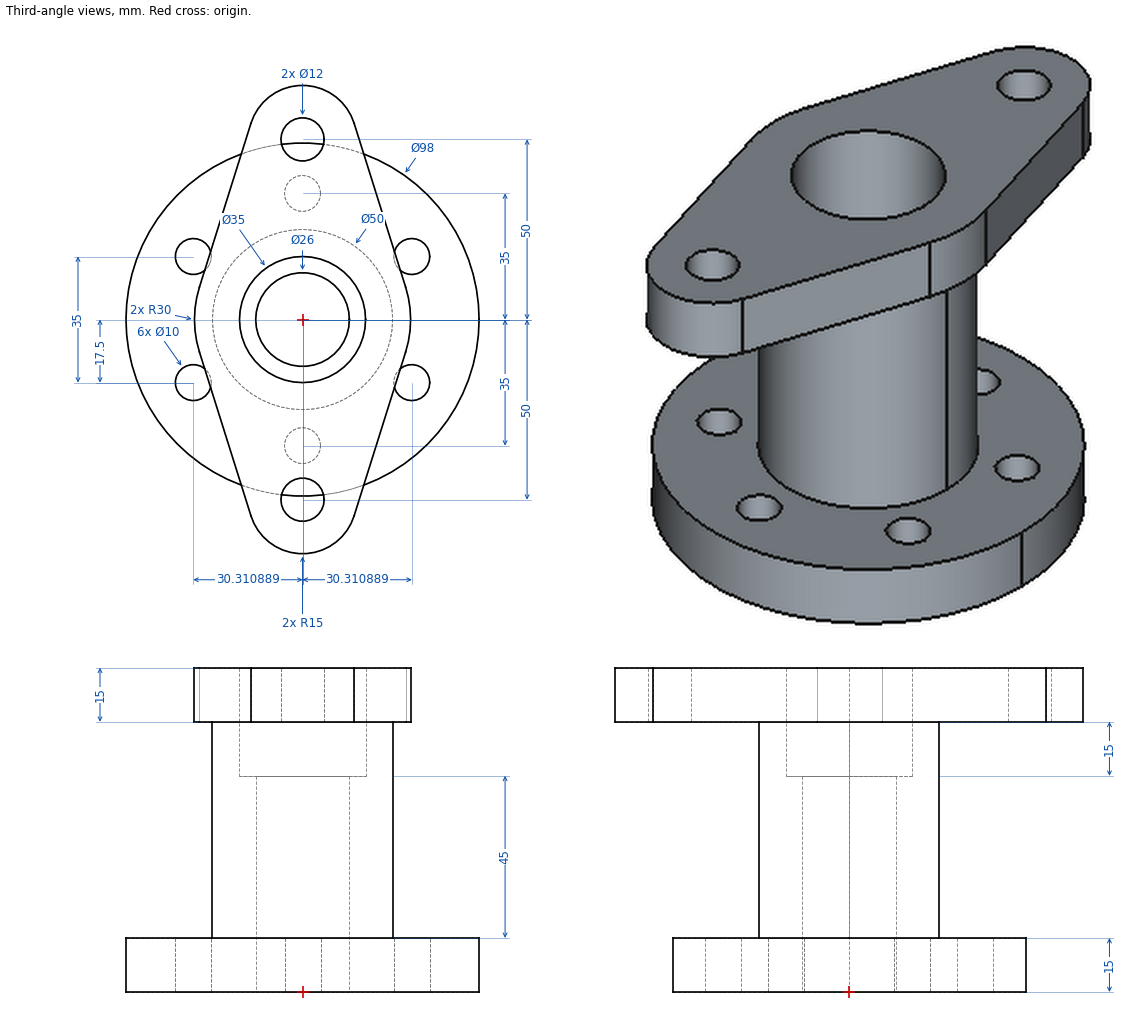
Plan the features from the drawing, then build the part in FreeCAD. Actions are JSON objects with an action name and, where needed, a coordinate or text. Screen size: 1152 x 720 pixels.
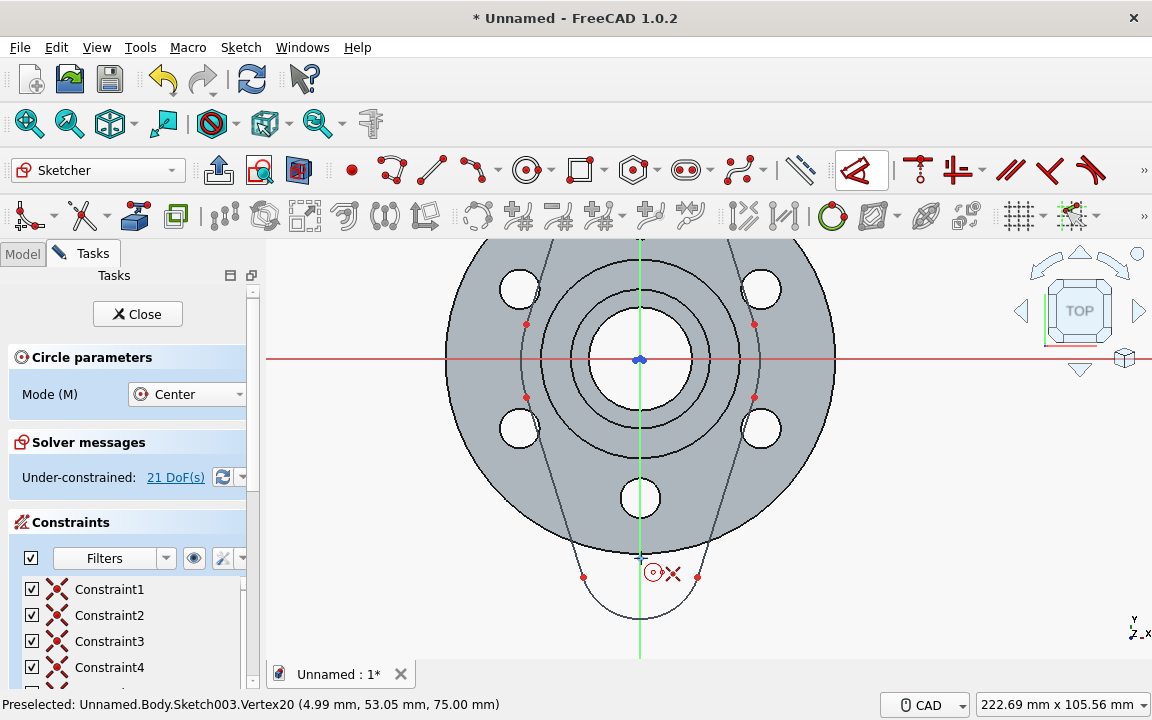
{"action": "left_click", "coordinate": [640, 558]}
{"action": "left_click", "coordinate": [657, 541]}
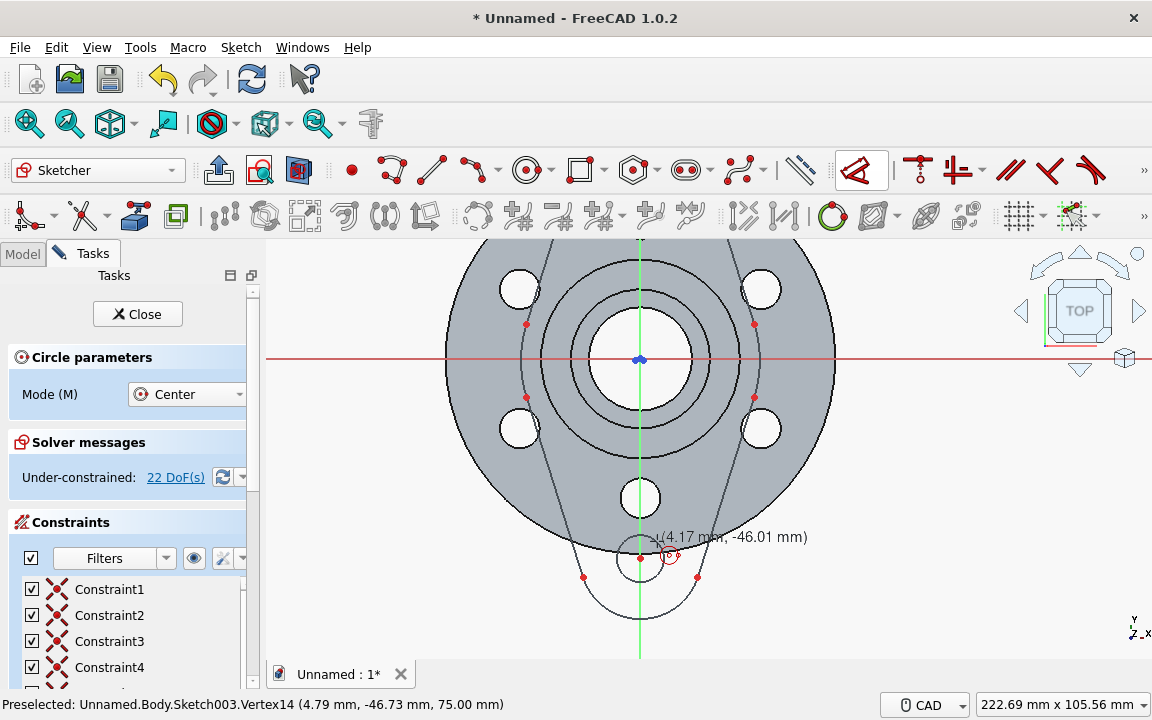
{"action": "left_click", "coordinate": [640, 359]}
{"action": "left_click", "coordinate": [690, 310]}
{"action": "key", "text": "Escape"}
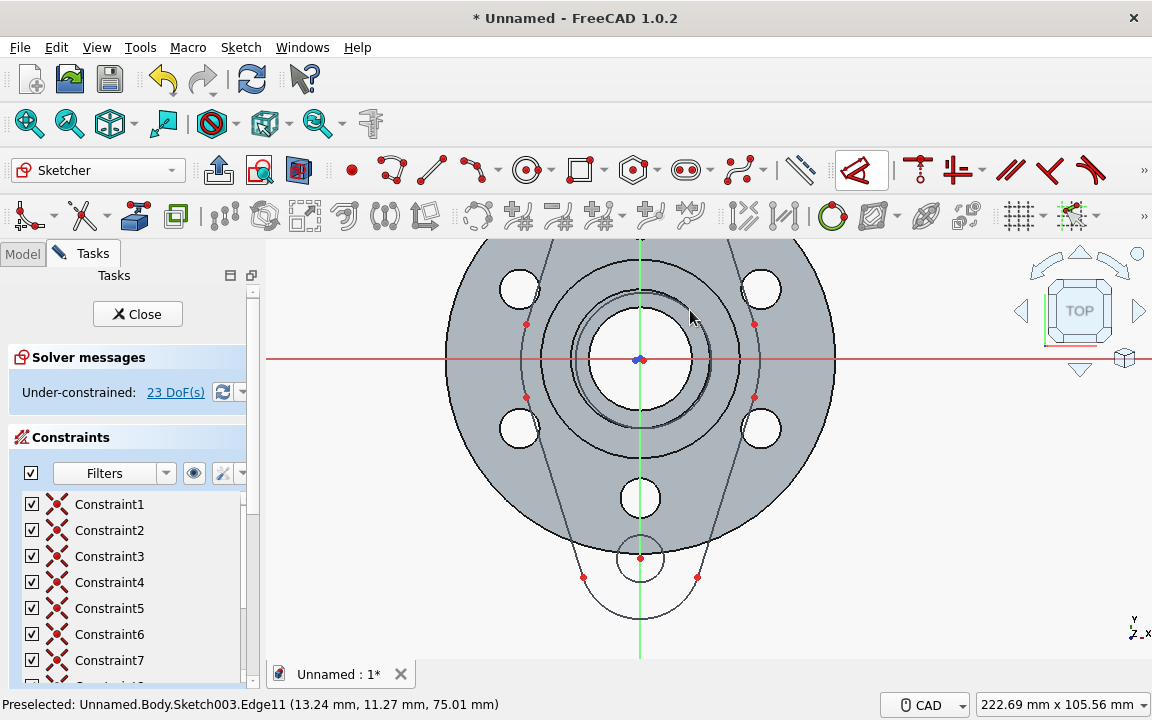
{"action": "left_click", "coordinate": [544, 270]}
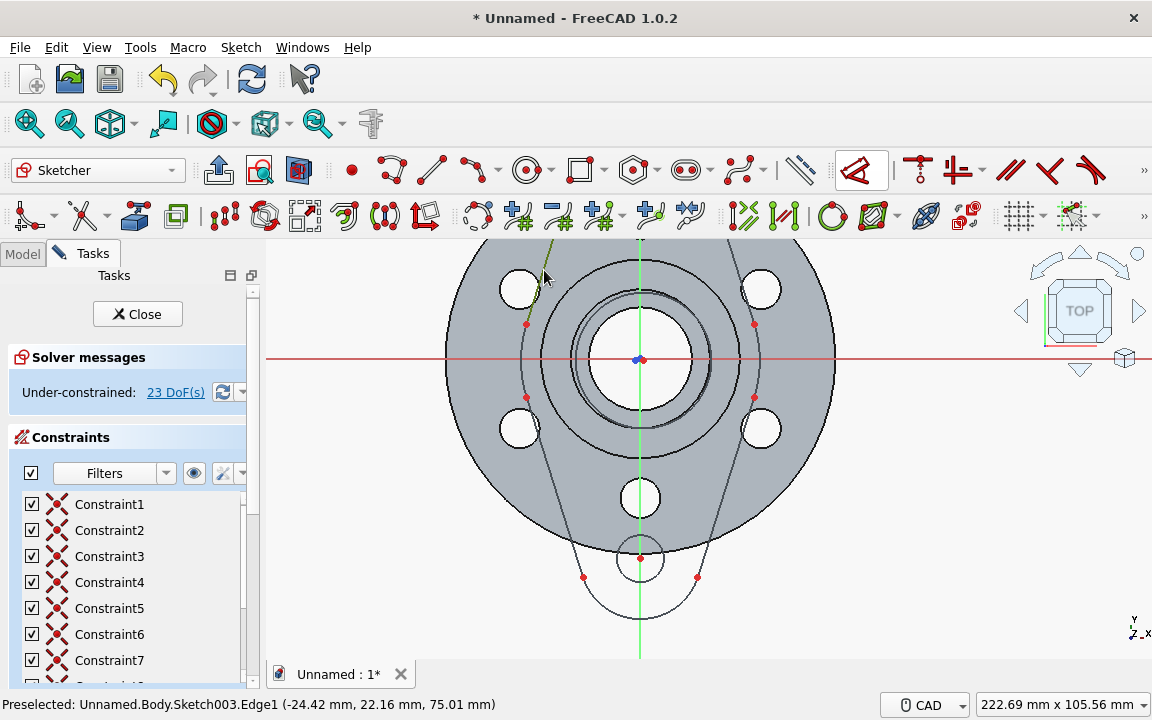
{"action": "left_click", "coordinate": [522, 346]}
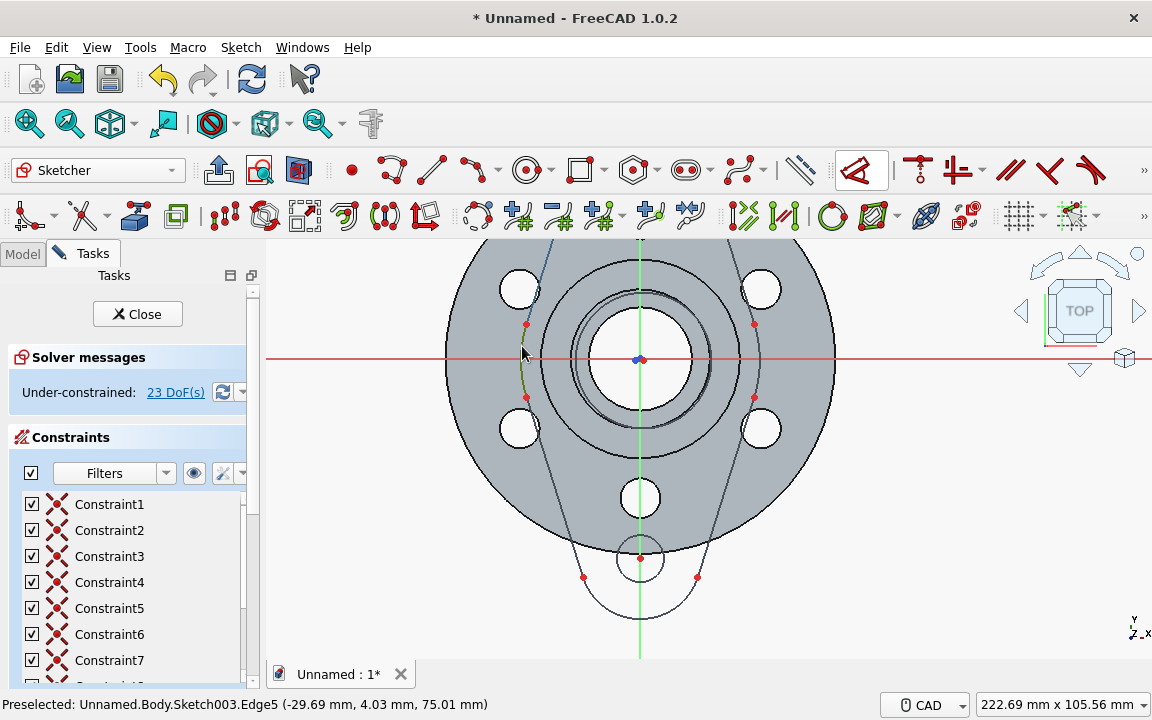
{"action": "key", "text": "t"}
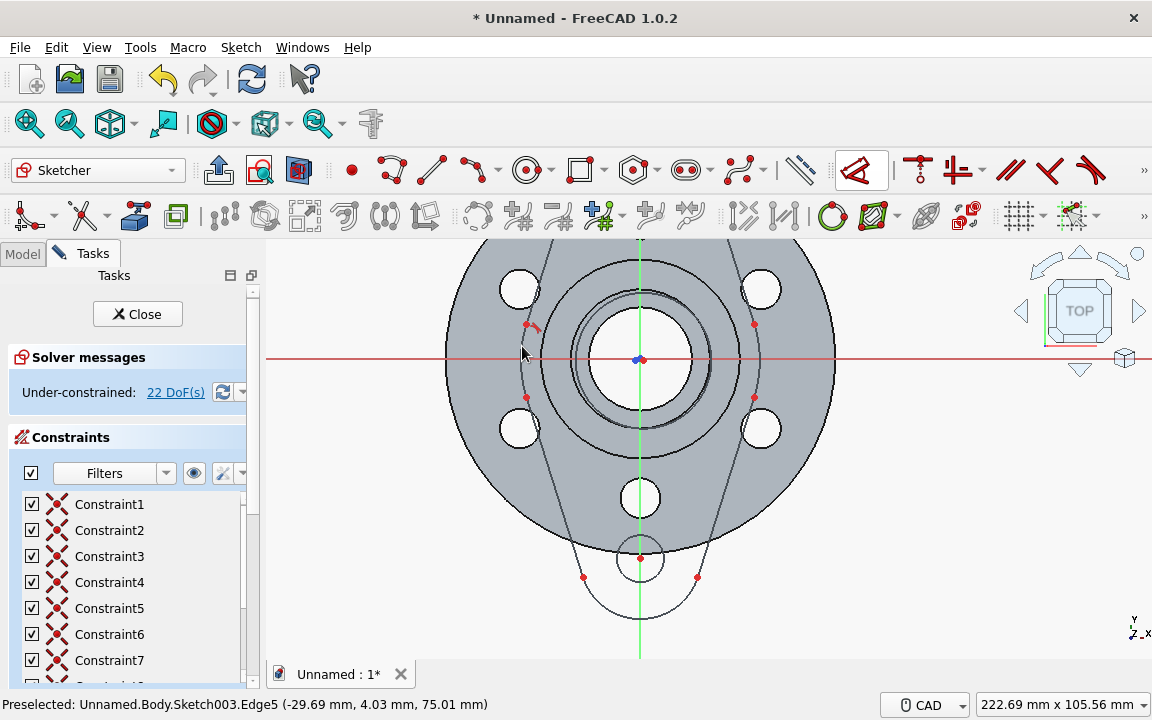
{"action": "left_click", "coordinate": [544, 270]}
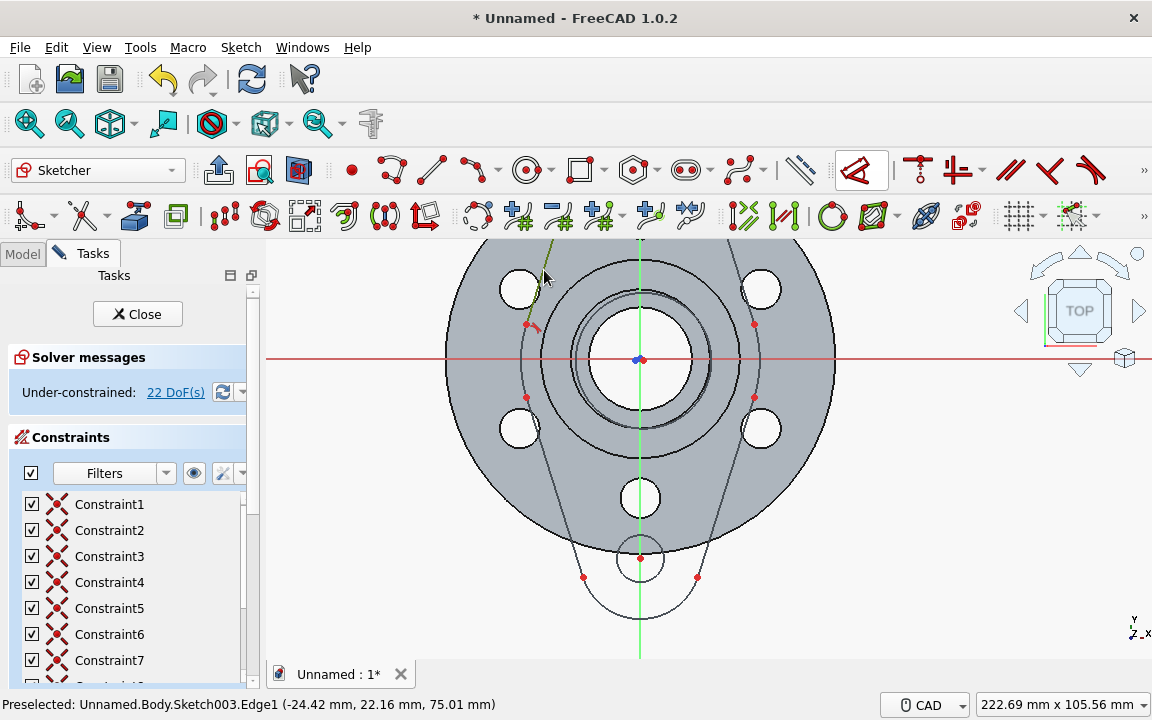
{"action": "scroll", "coordinate": [641, 559], "scroll_direction": "down", "scroll_amount": 3}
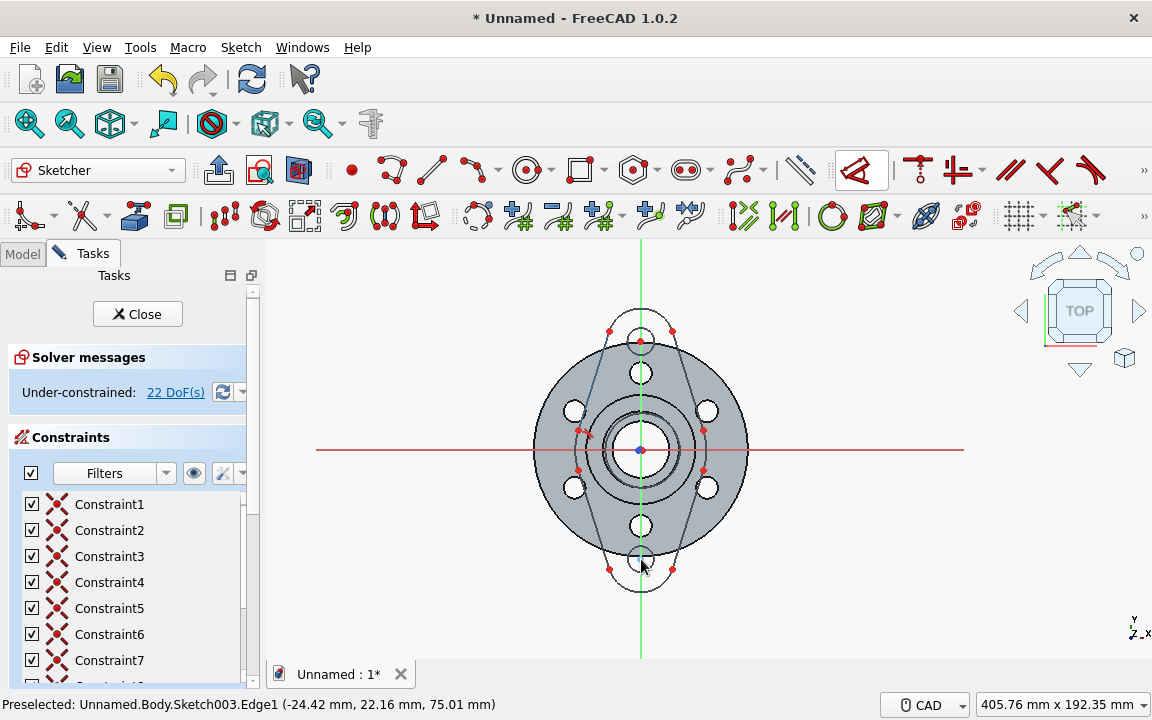
{"action": "left_click", "coordinate": [657, 313]}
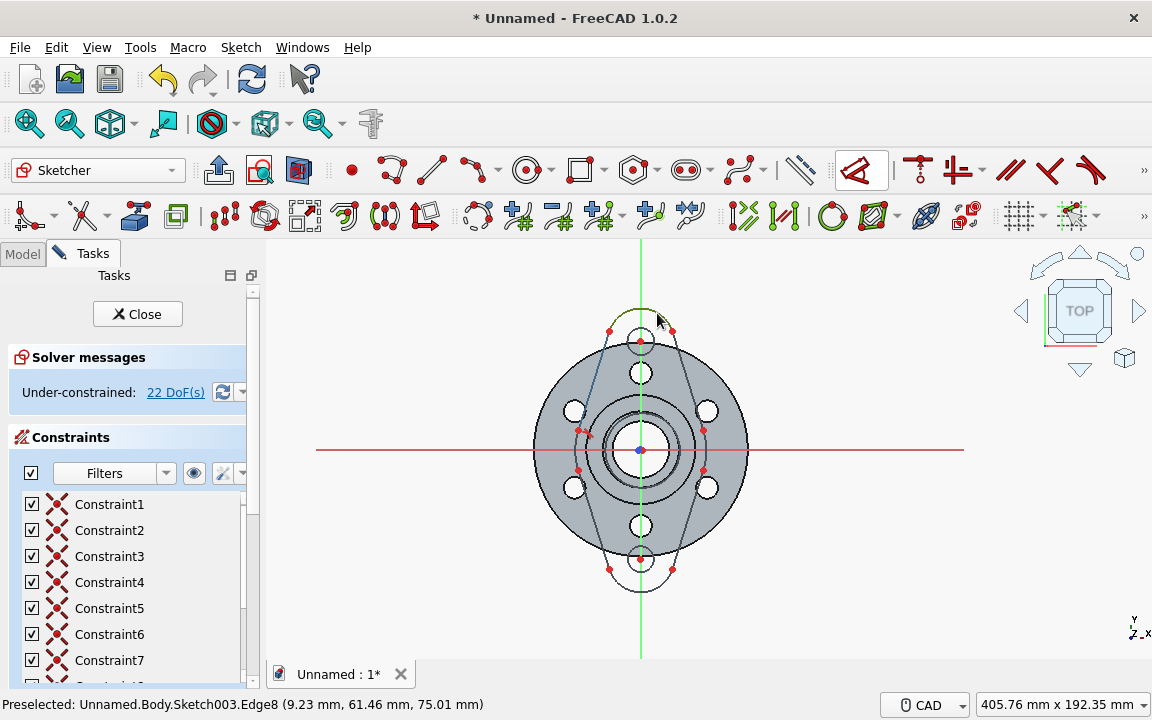
{"action": "key", "text": "t"}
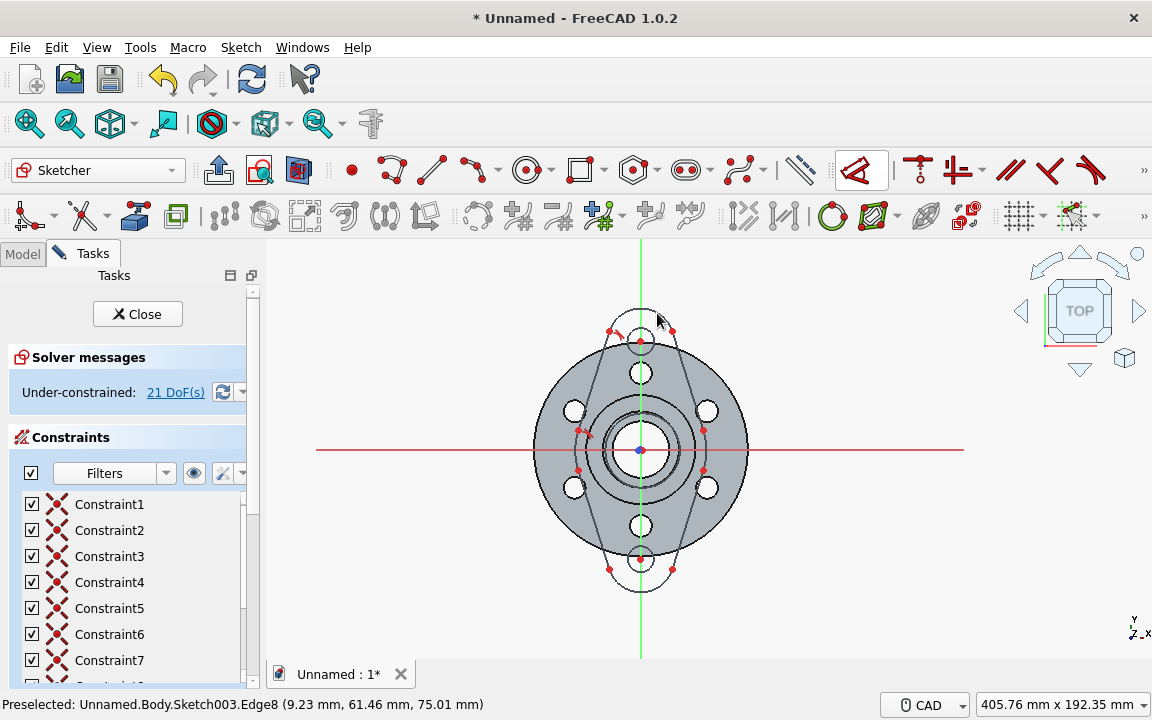
{"action": "left_click", "coordinate": [588, 500]}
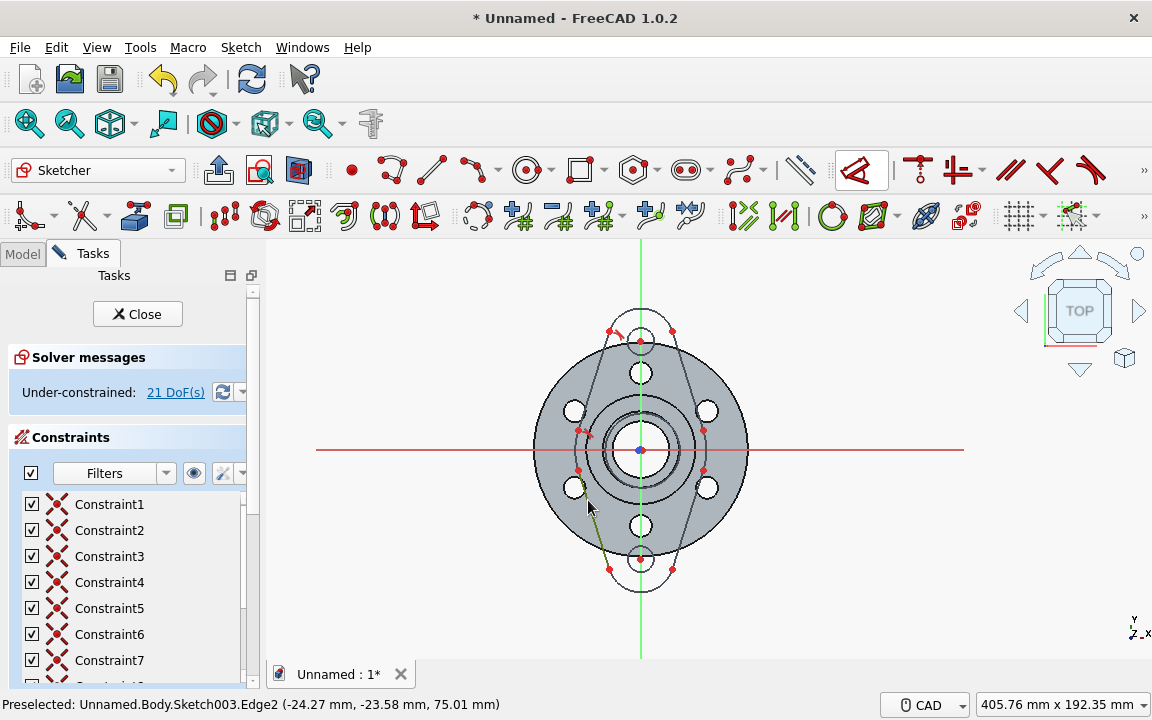
{"action": "scroll", "coordinate": [576, 459], "scroll_direction": "up", "scroll_amount": 3}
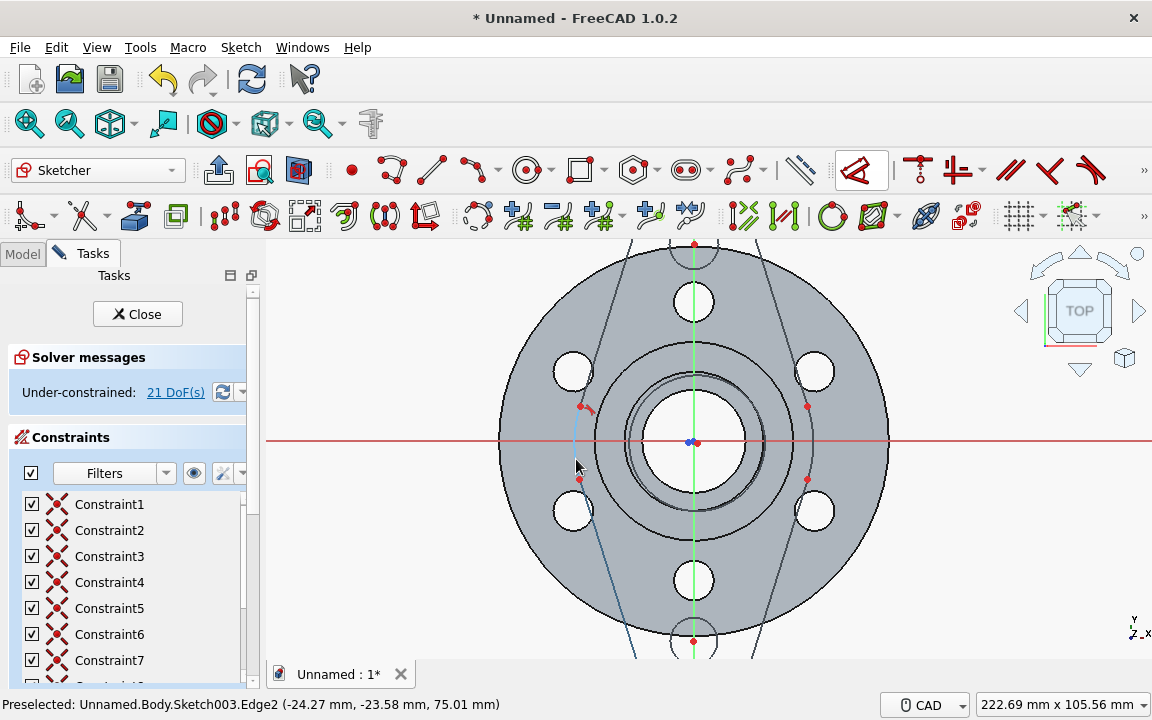
{"action": "left_click", "coordinate": [575, 458]}